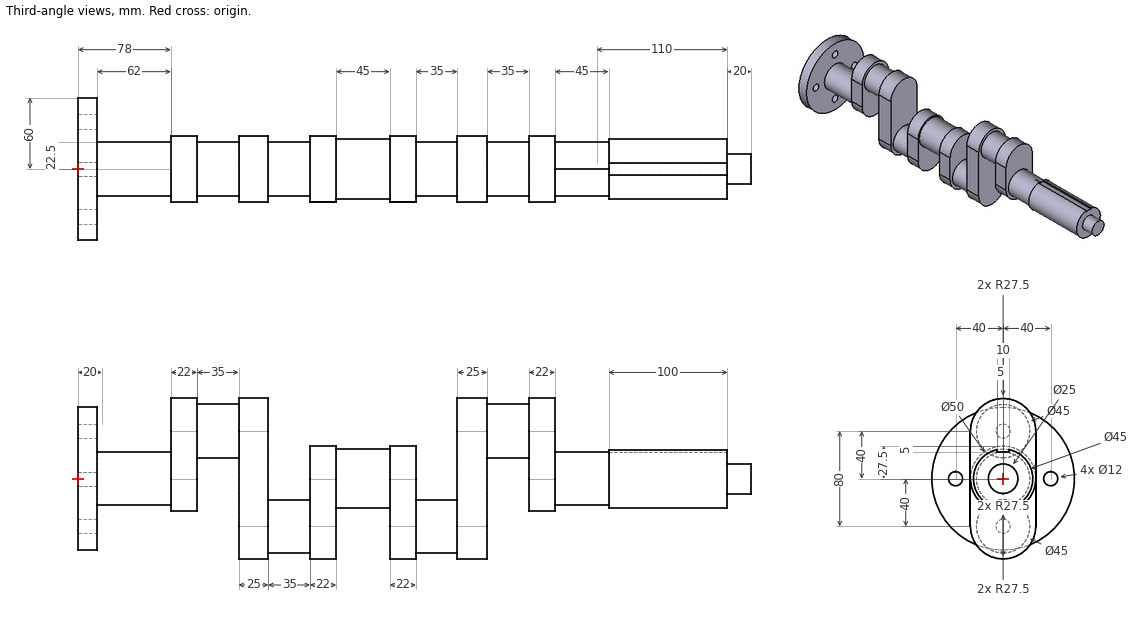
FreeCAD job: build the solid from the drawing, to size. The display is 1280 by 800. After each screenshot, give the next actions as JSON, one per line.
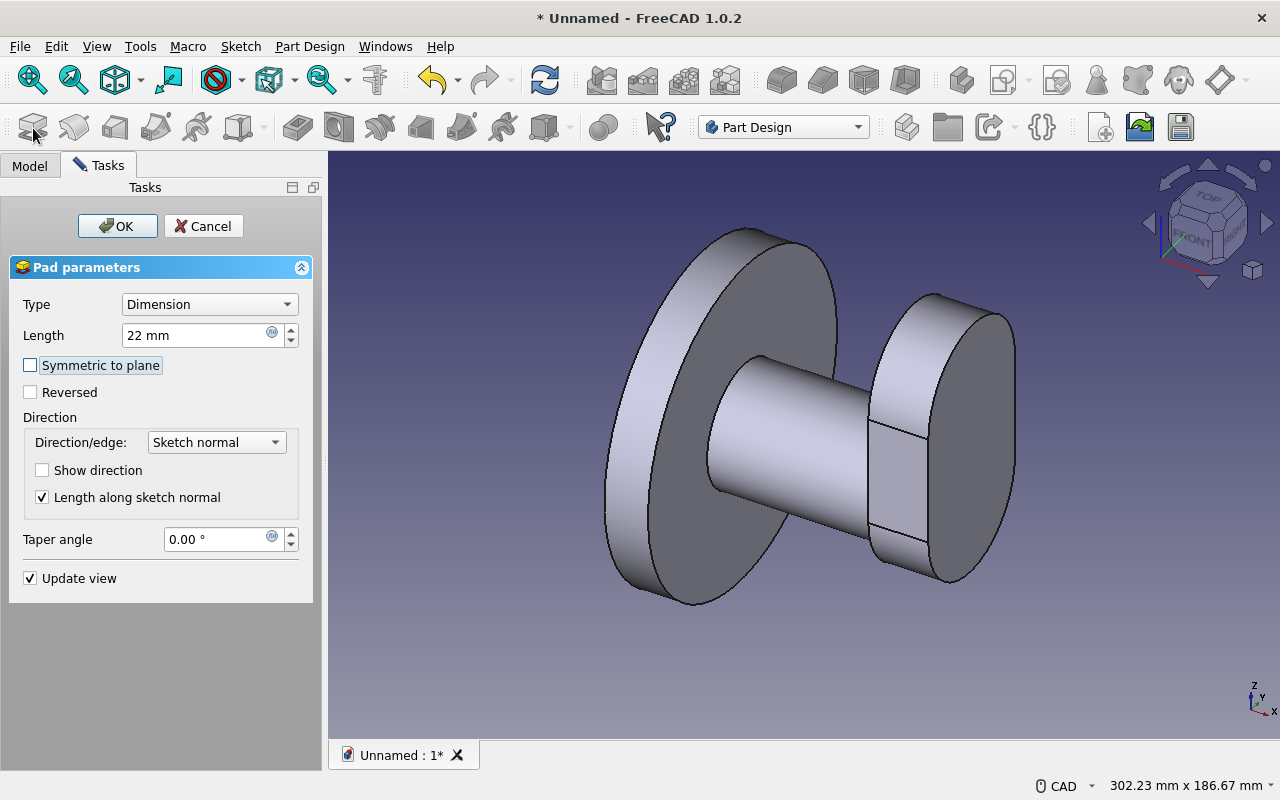
{"action": "left_click", "coordinate": [118, 226]}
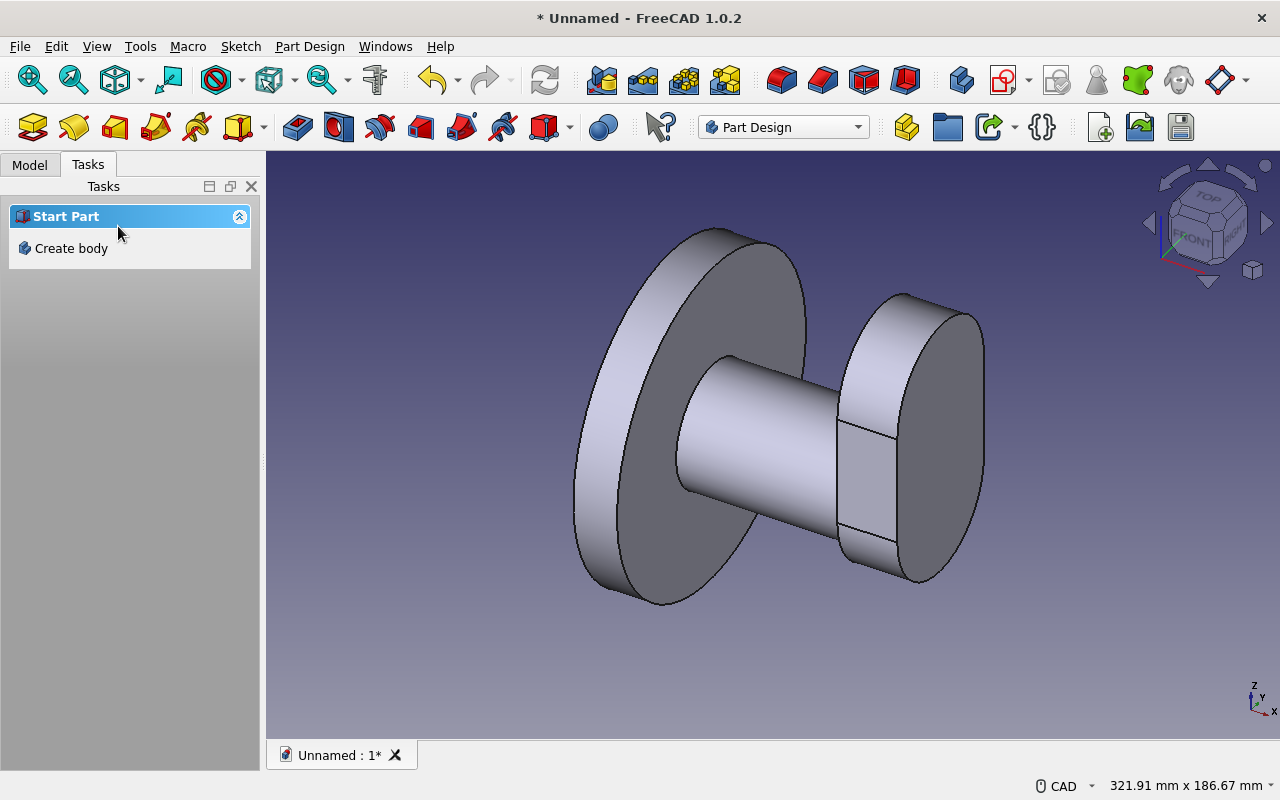
{"action": "left_click", "coordinate": [33, 80]}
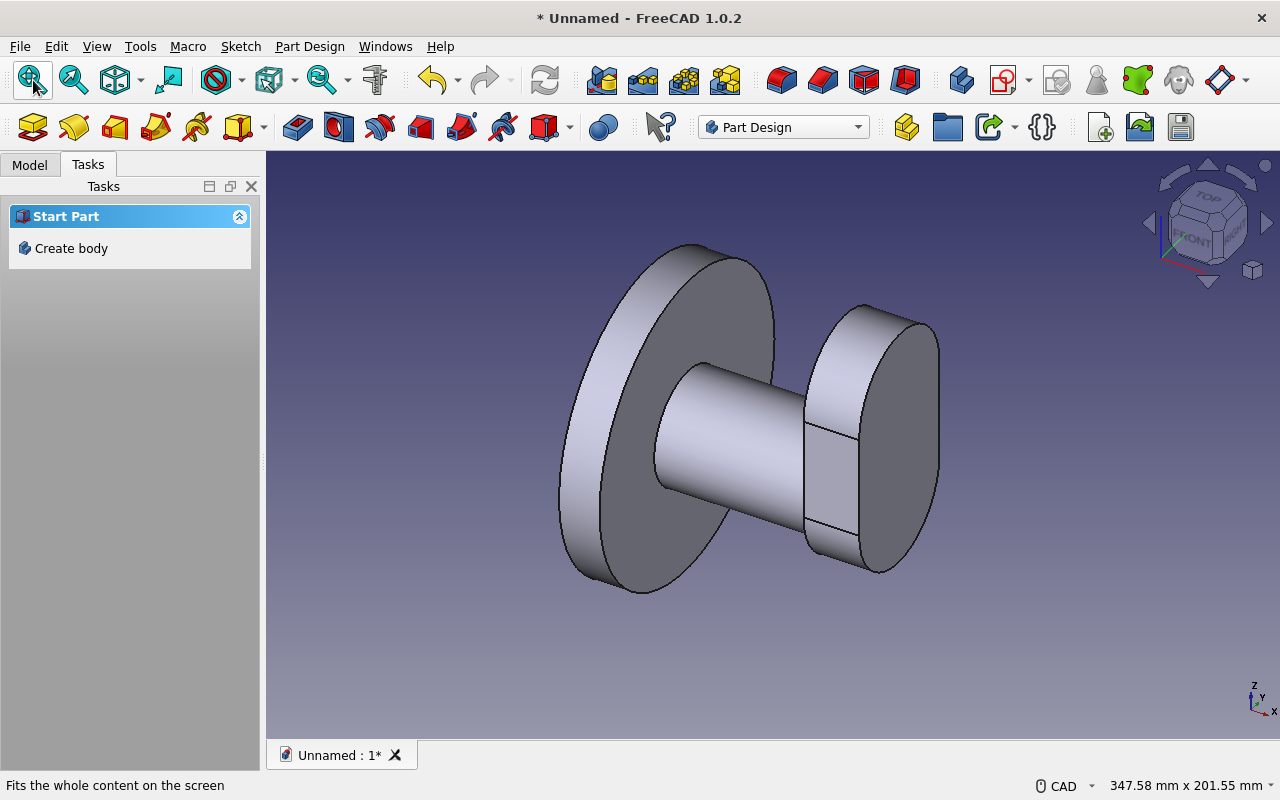
{"action": "left_click", "coordinate": [899, 415]}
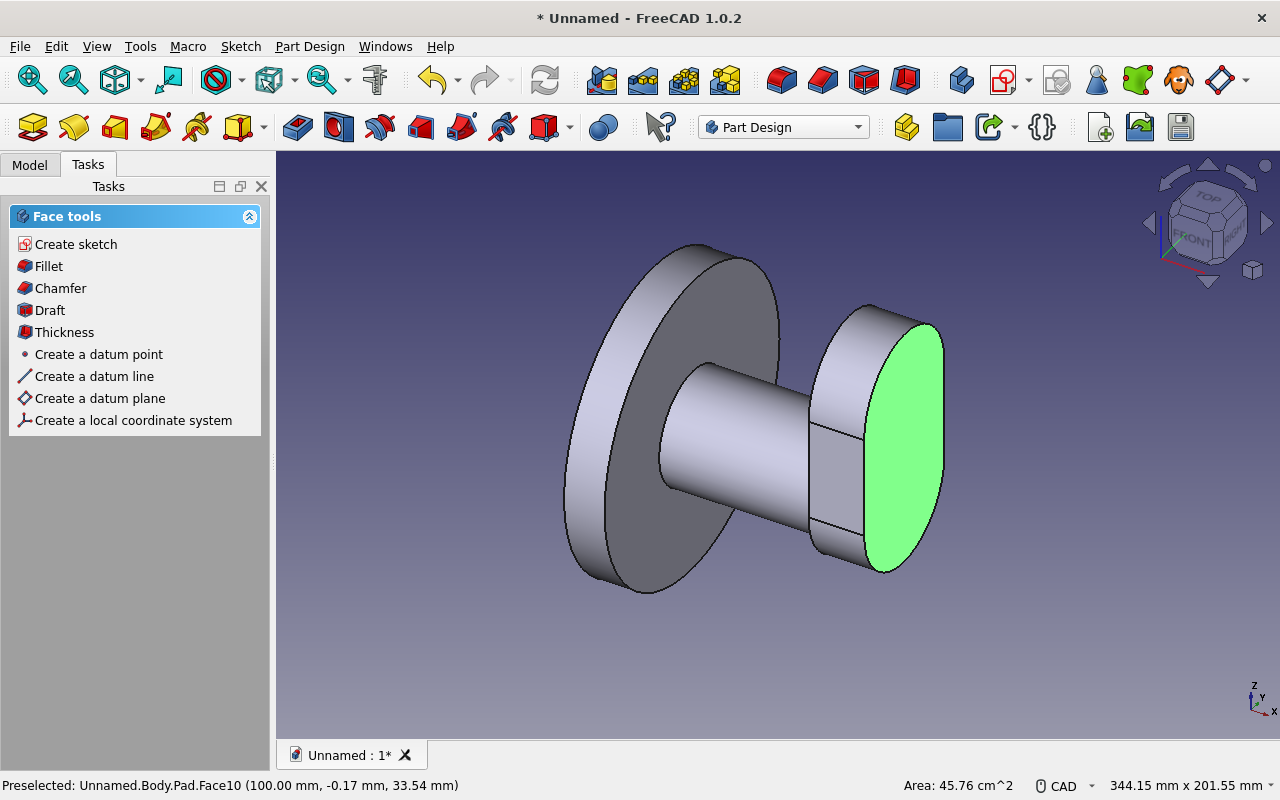
{"action": "left_click", "coordinate": [1002, 80]}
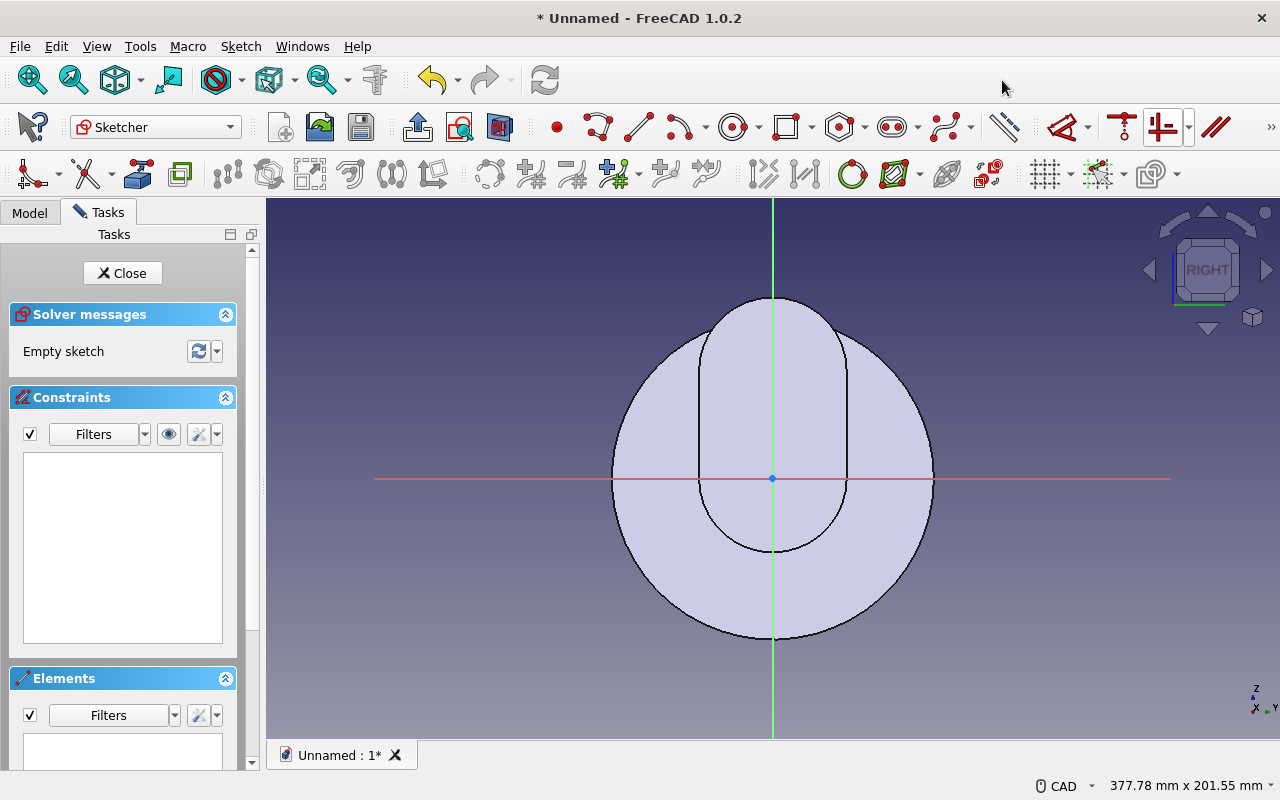
{"action": "scroll", "coordinate": [829, 335], "scroll_direction": "up", "scroll_amount": 4}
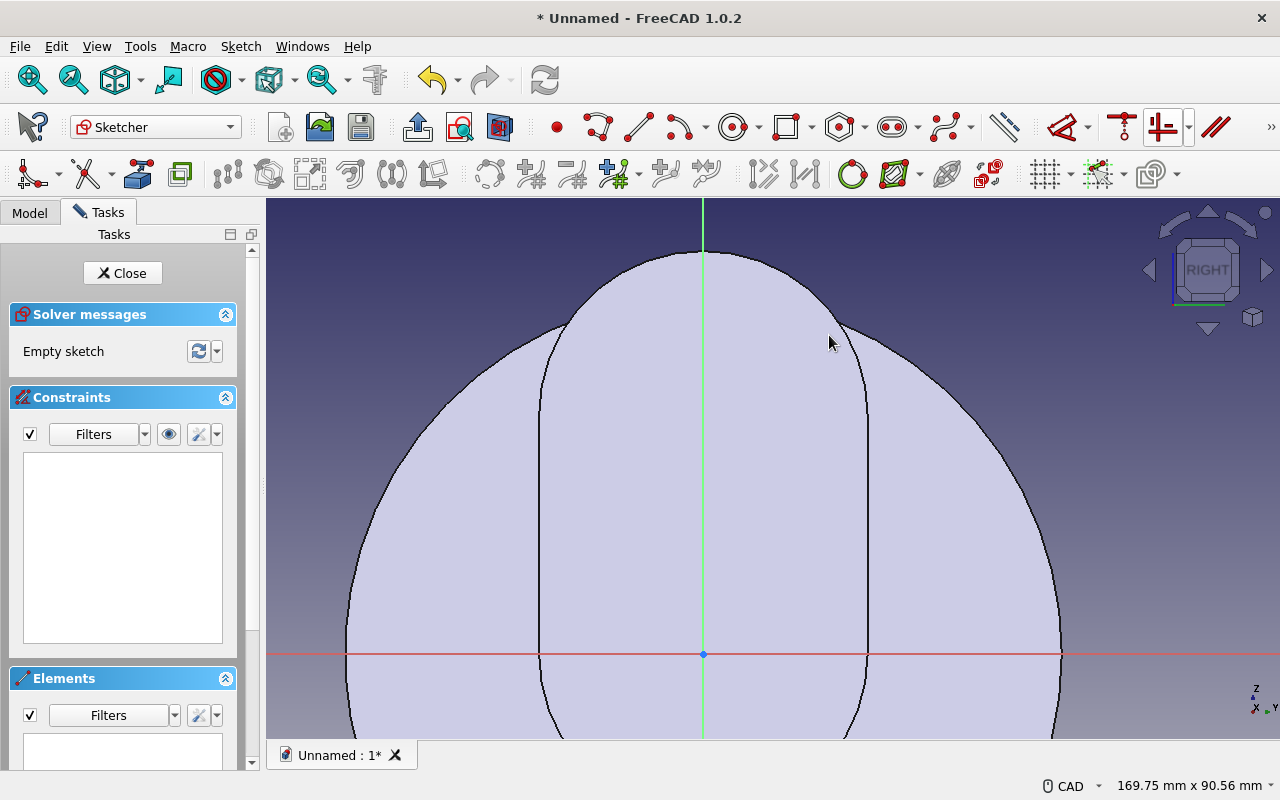
{"action": "left_click", "coordinate": [732, 128]}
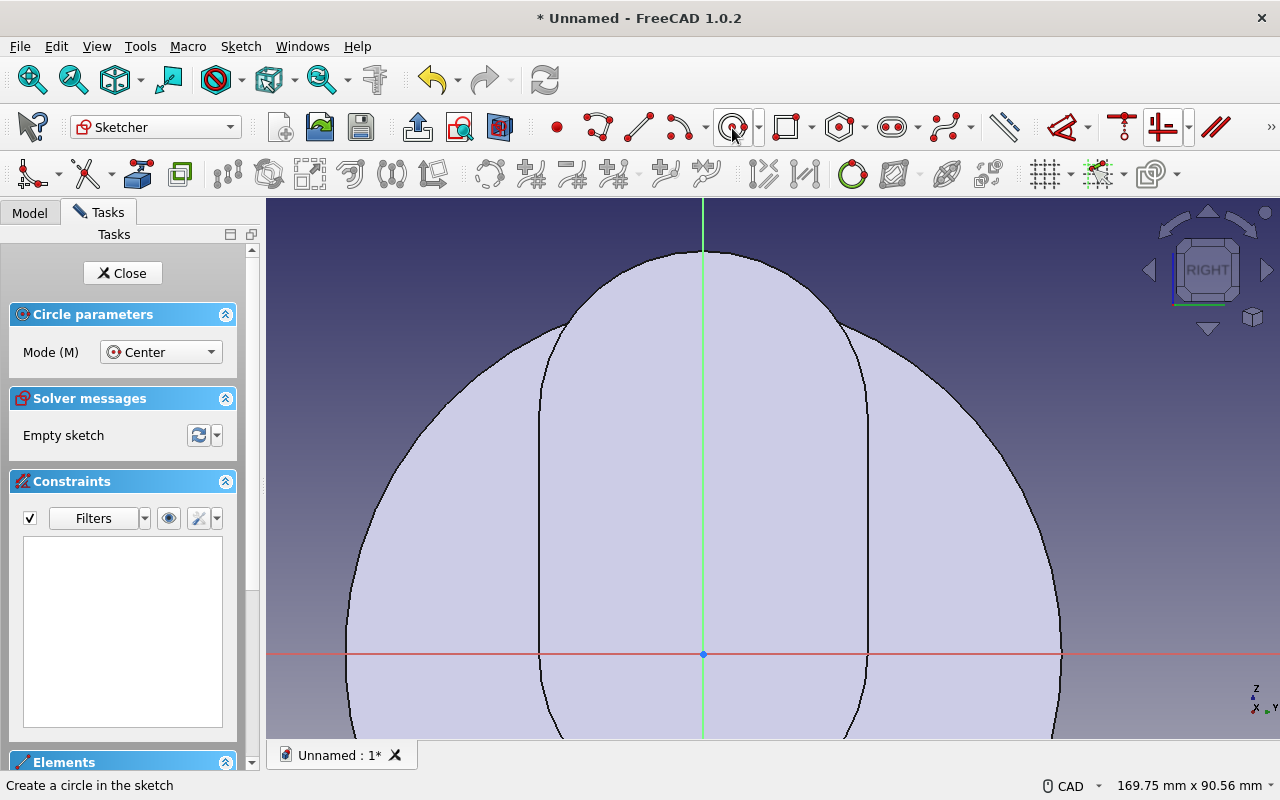
{"action": "left_click", "coordinate": [703, 415]}
{"action": "left_click", "coordinate": [798, 320]}
{"action": "key", "text": "Escape"}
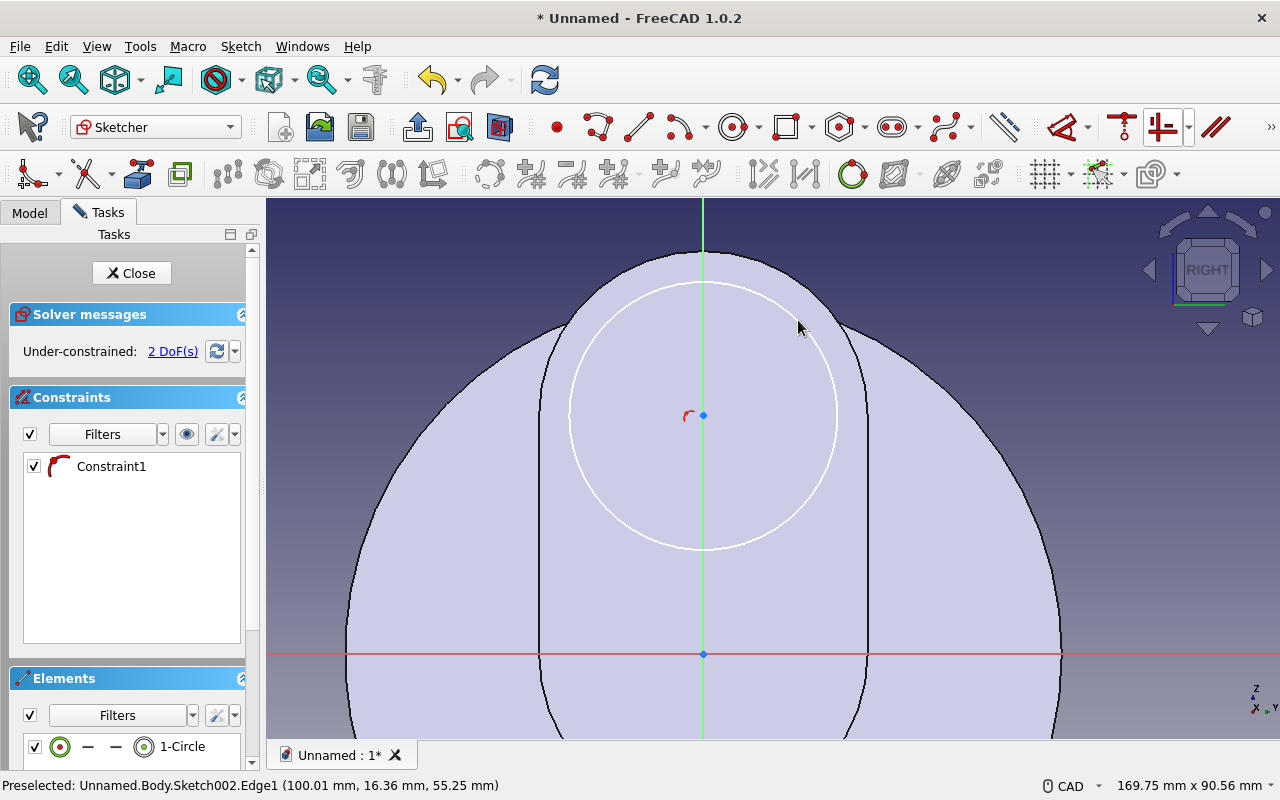
{"action": "left_click", "coordinate": [1062, 128]}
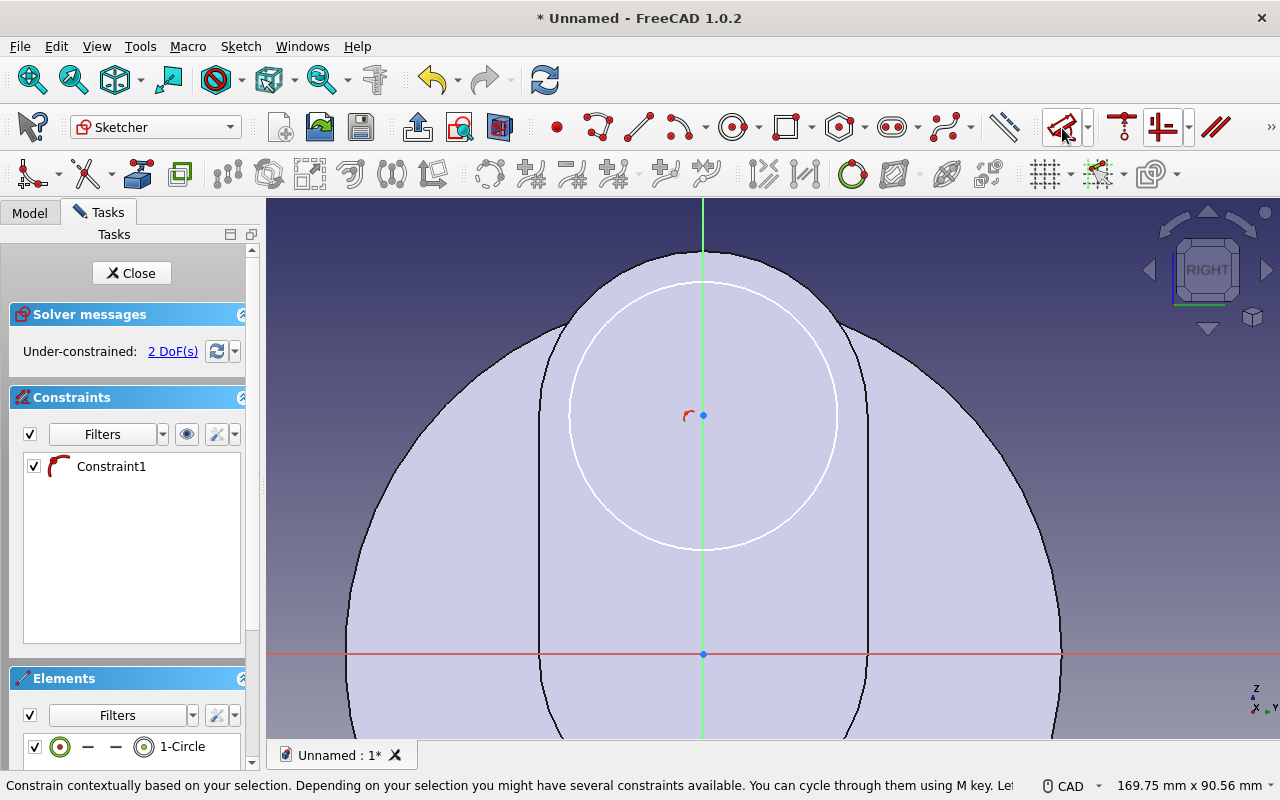
{"action": "left_click", "coordinate": [798, 321]}
{"action": "left_click", "coordinate": [821, 298]}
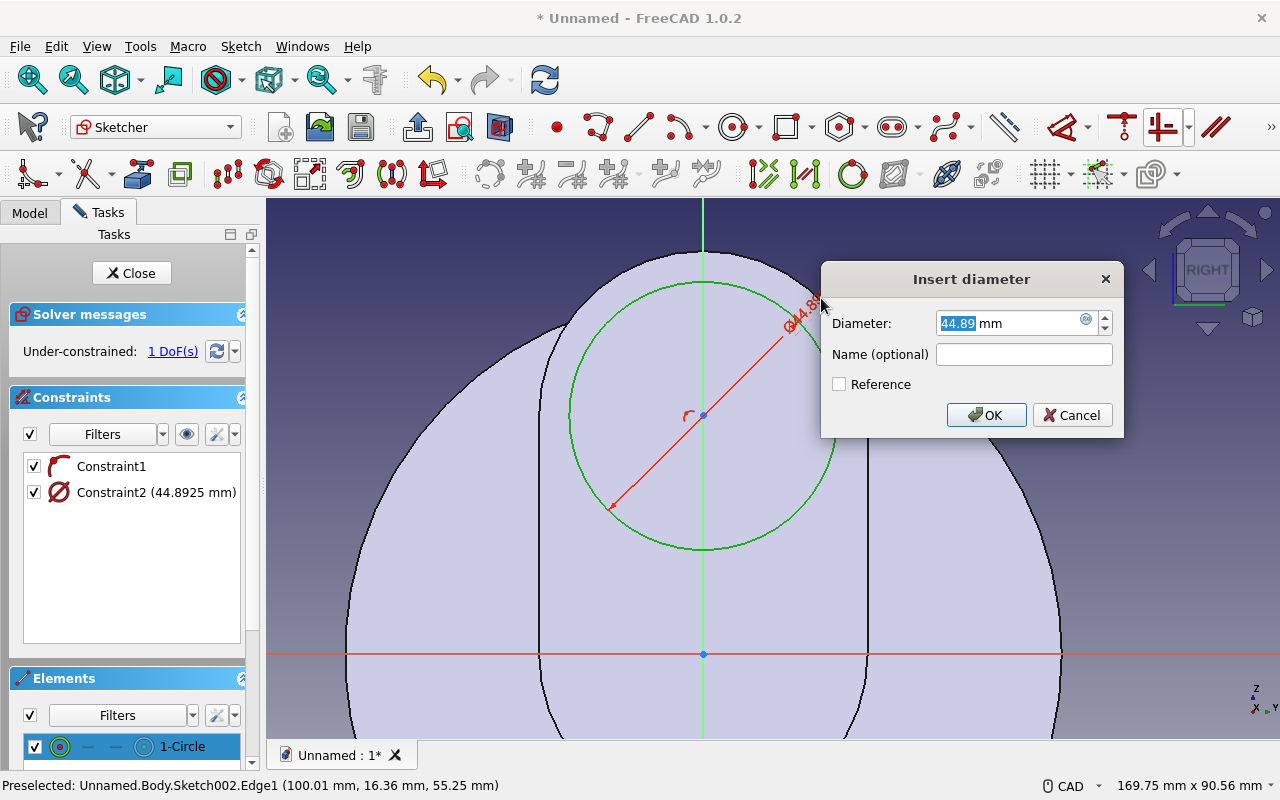
{"action": "type", "text": "45"}
{"action": "key", "text": "Return"}